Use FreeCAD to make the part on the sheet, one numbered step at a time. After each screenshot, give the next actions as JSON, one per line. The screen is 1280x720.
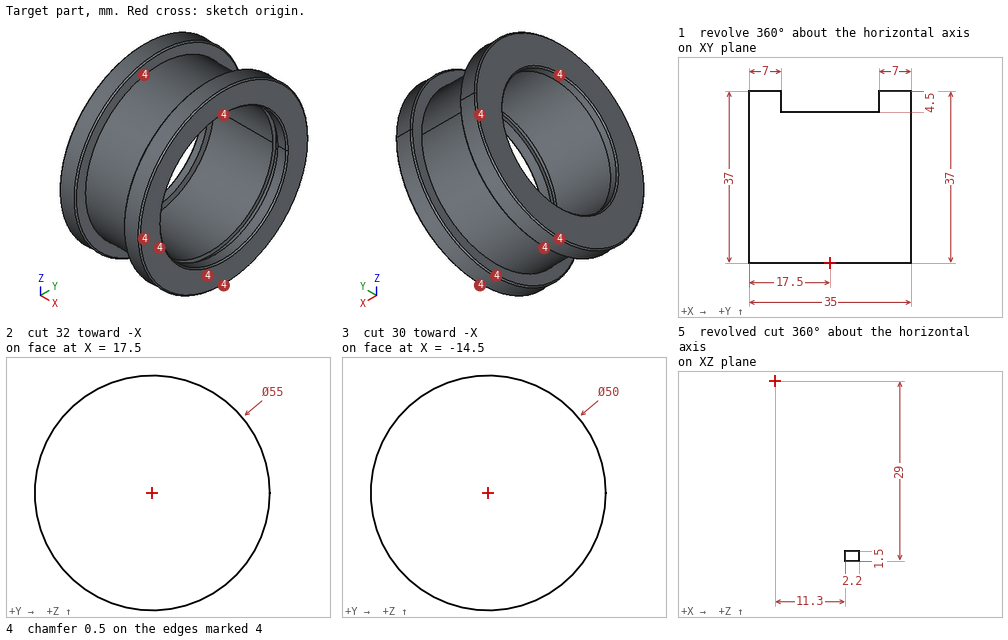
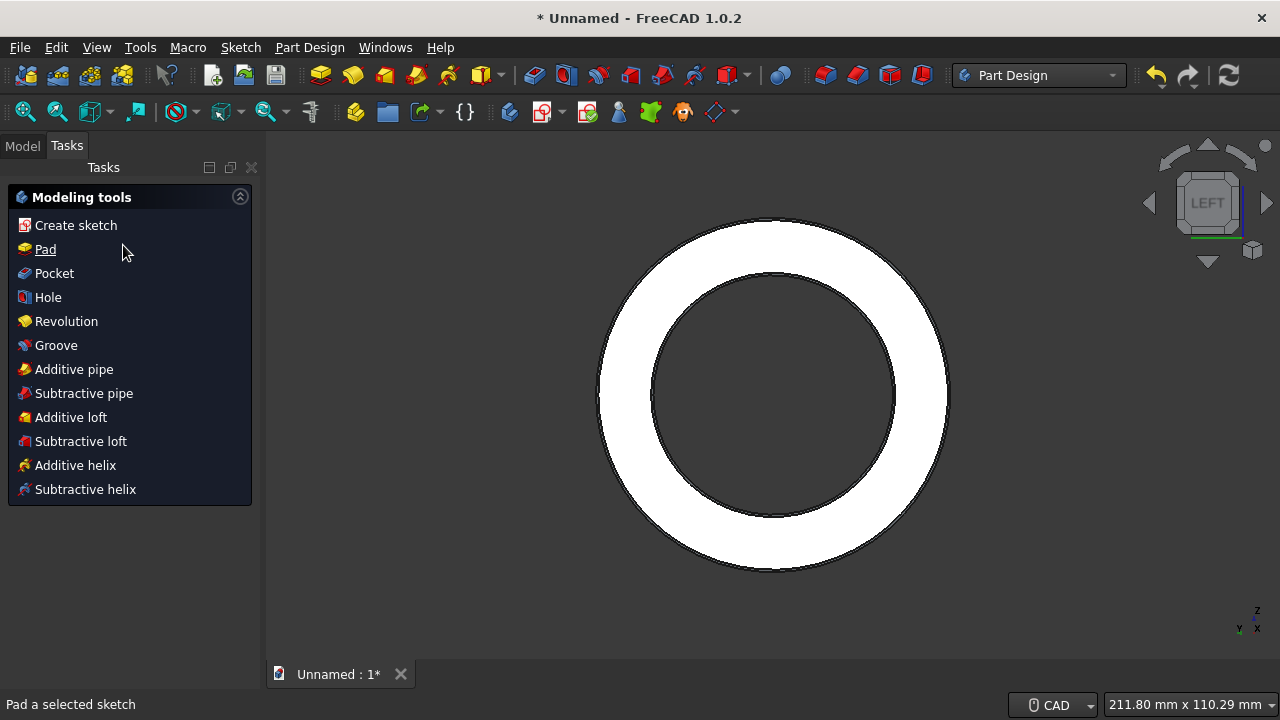
{"action": "left_click", "coordinate": [600, 76]}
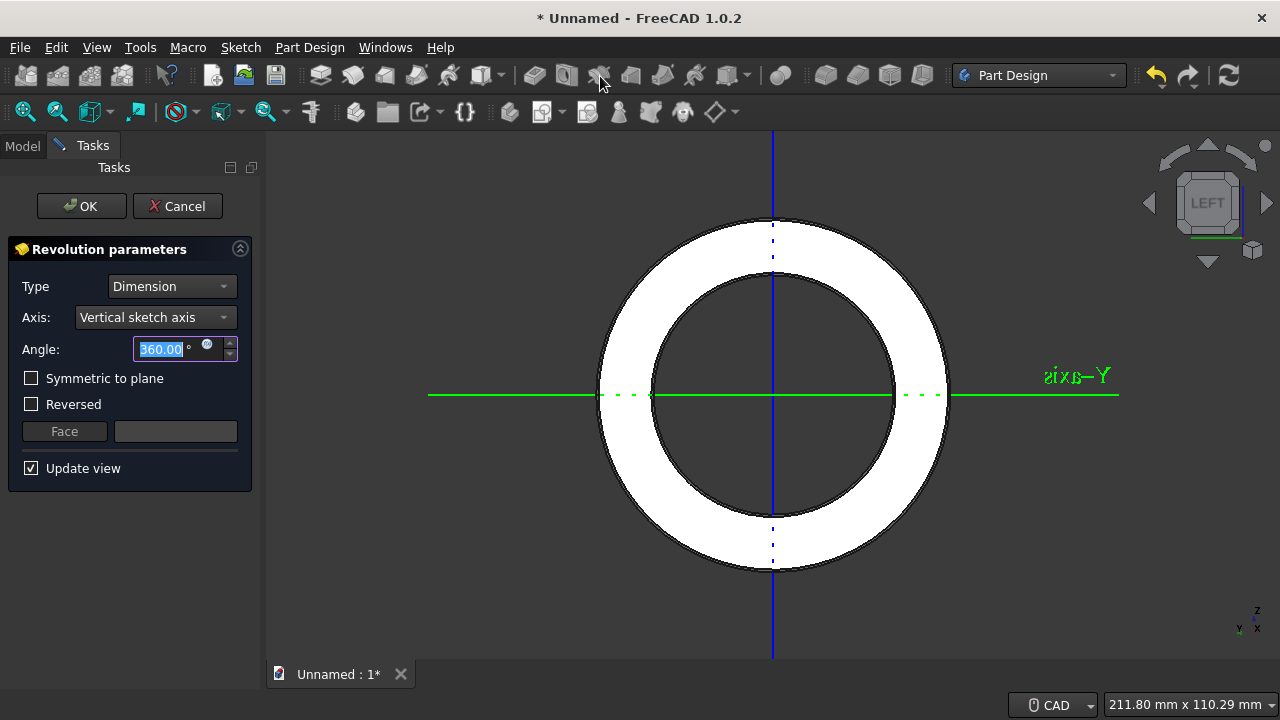
{"action": "left_click", "coordinate": [156, 318]}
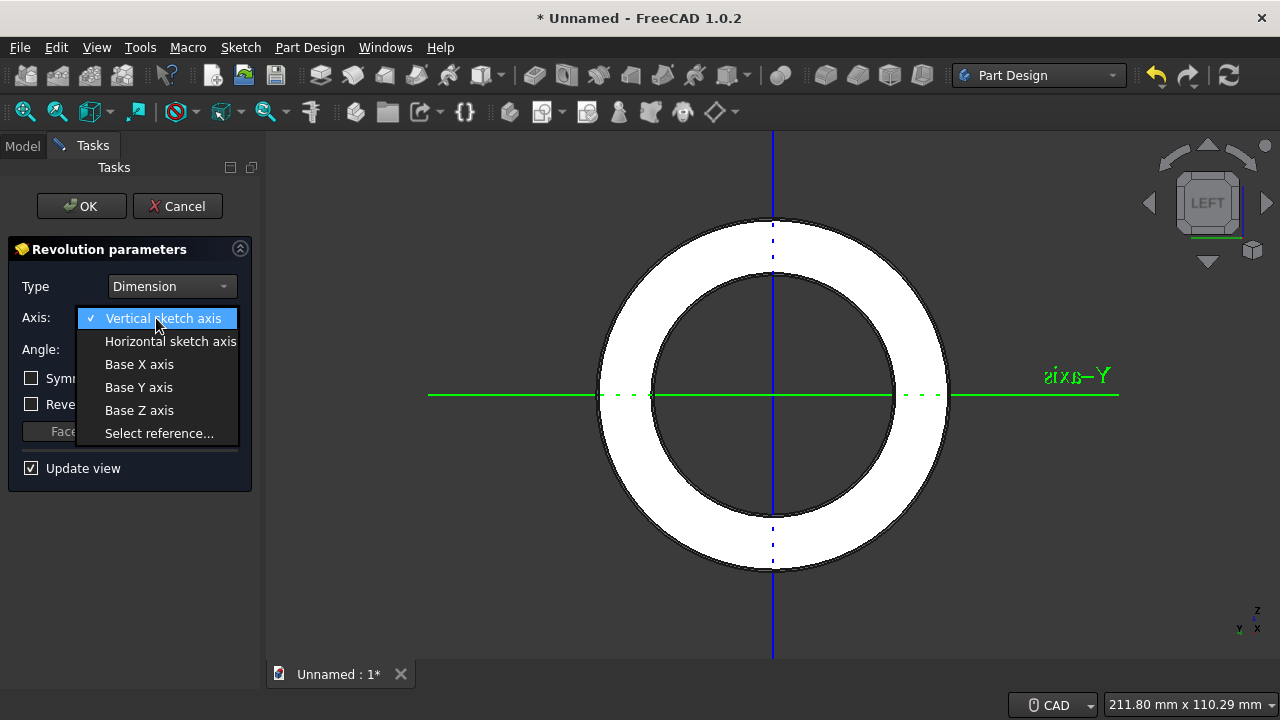
{"action": "left_click", "coordinate": [156, 342]}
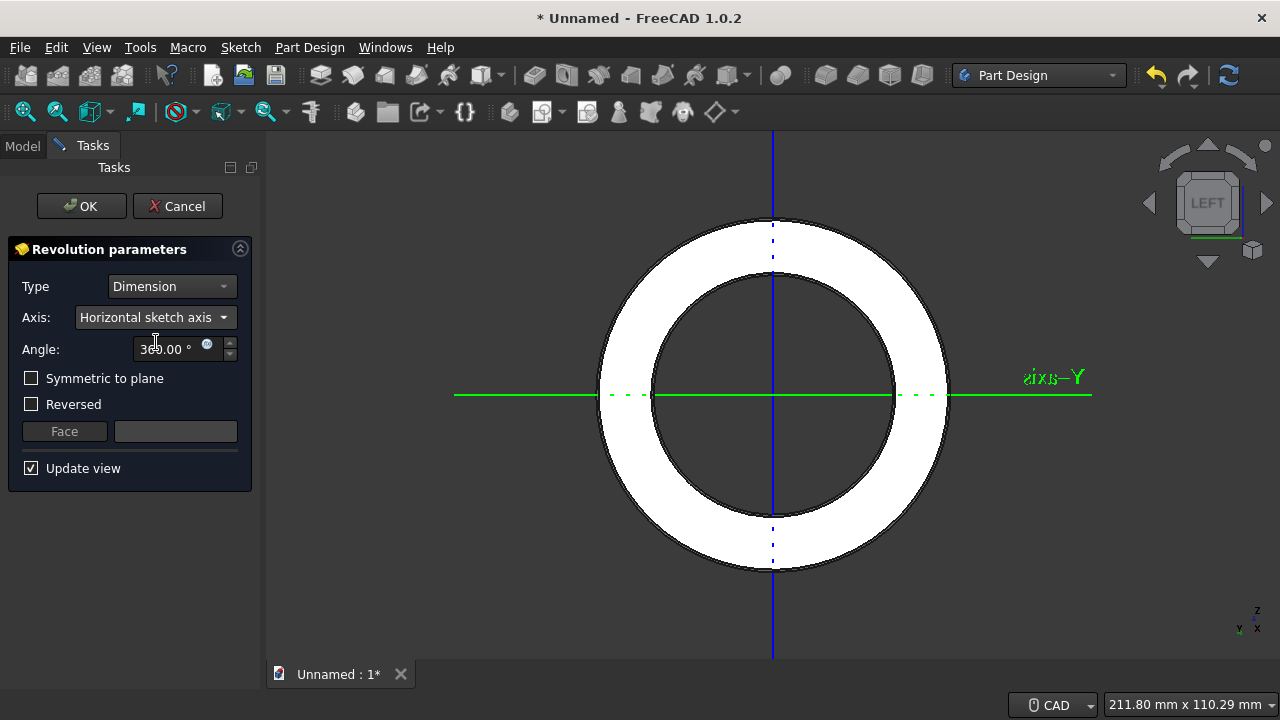
{"action": "left_click", "coordinate": [82, 206]}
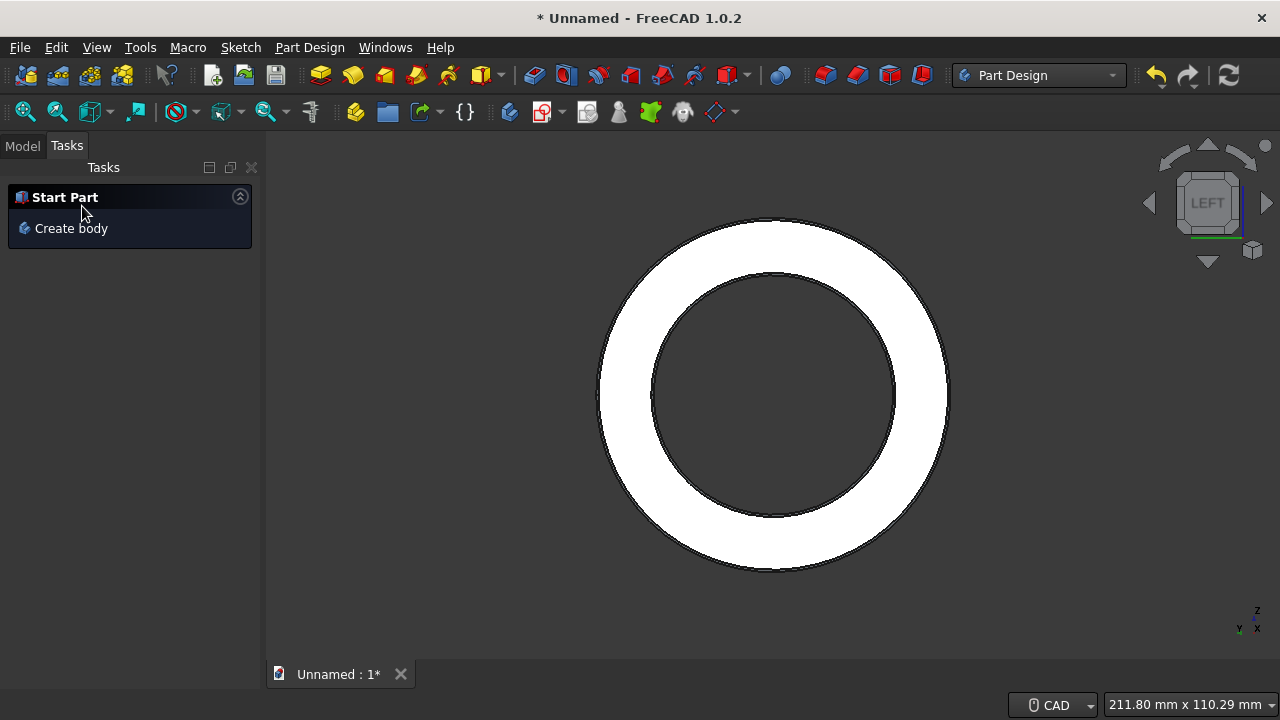
{"action": "key", "text": "0"}